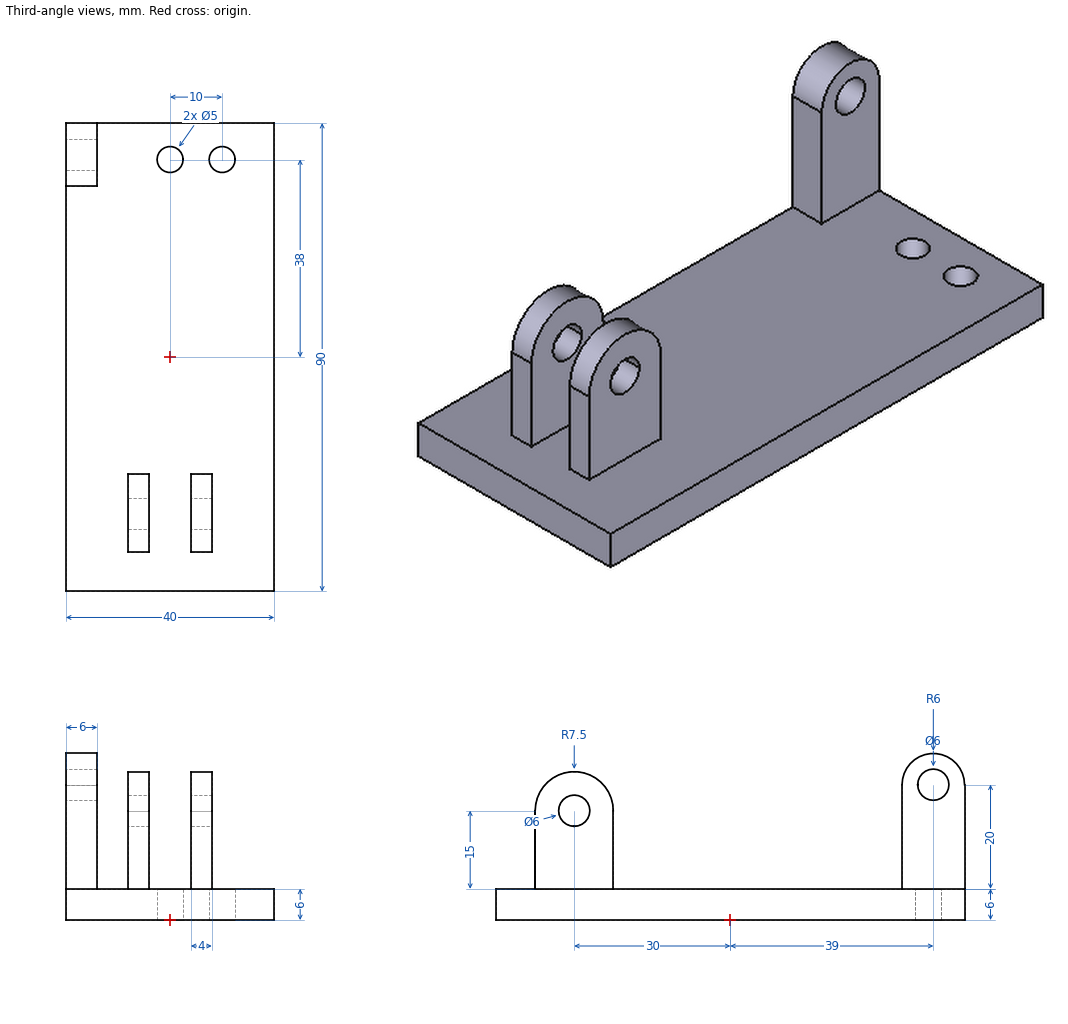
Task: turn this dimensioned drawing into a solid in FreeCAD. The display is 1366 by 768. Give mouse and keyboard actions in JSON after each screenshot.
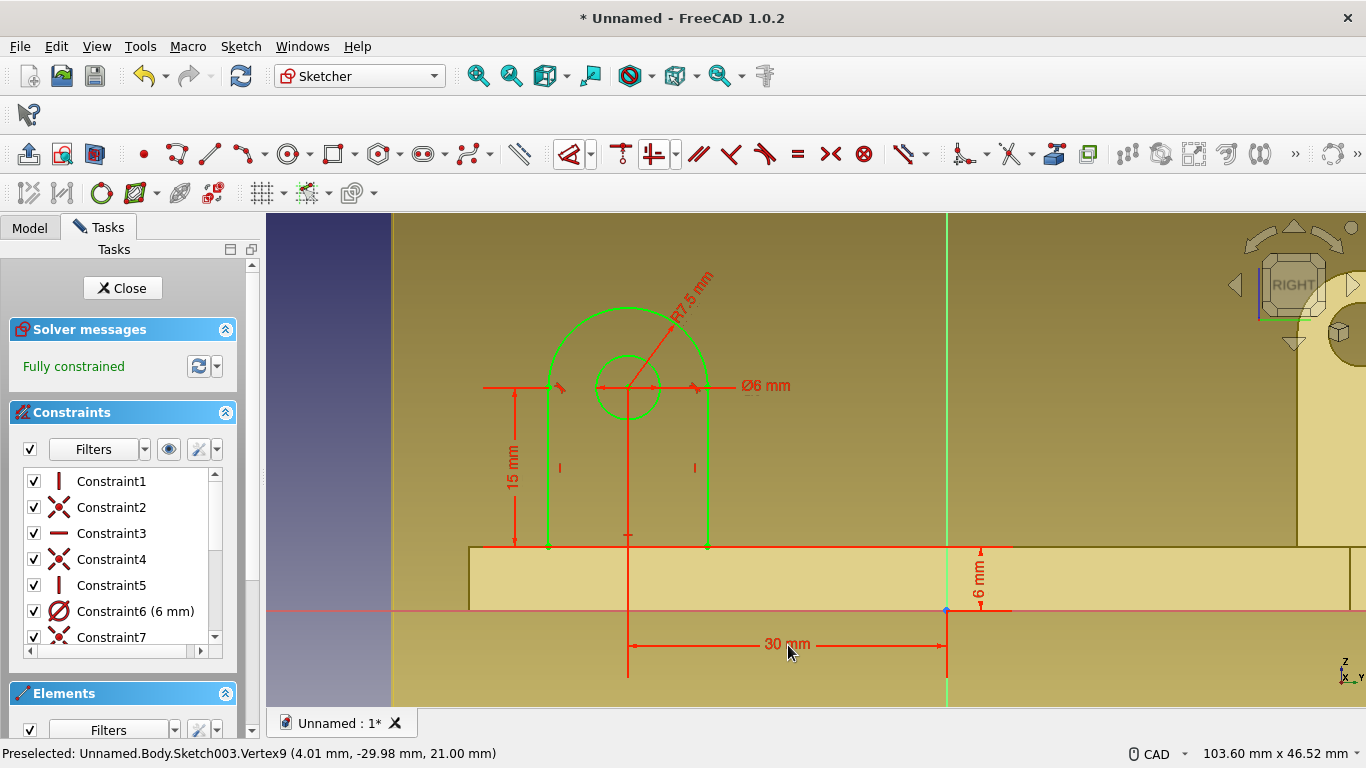
{"action": "left_click", "coordinate": [123, 288]}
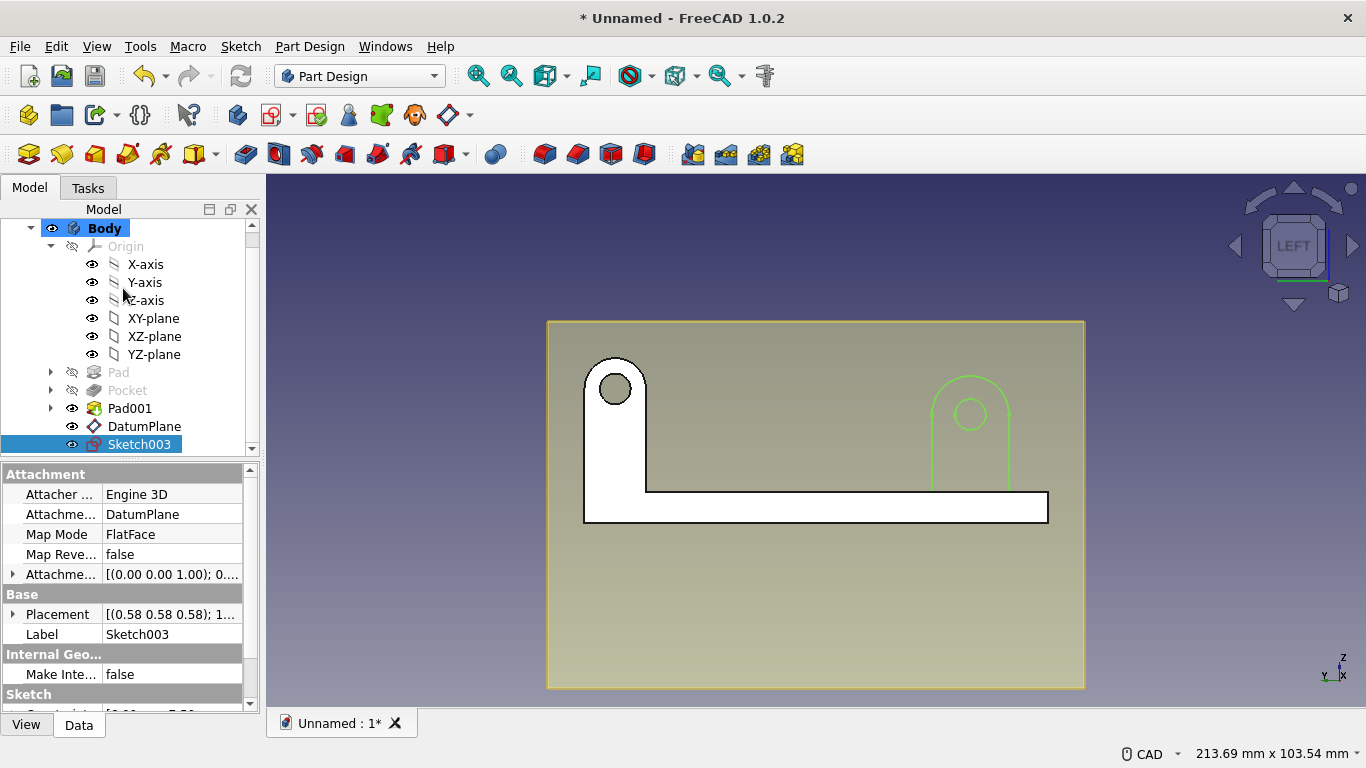
{"action": "left_click", "coordinate": [29, 154]}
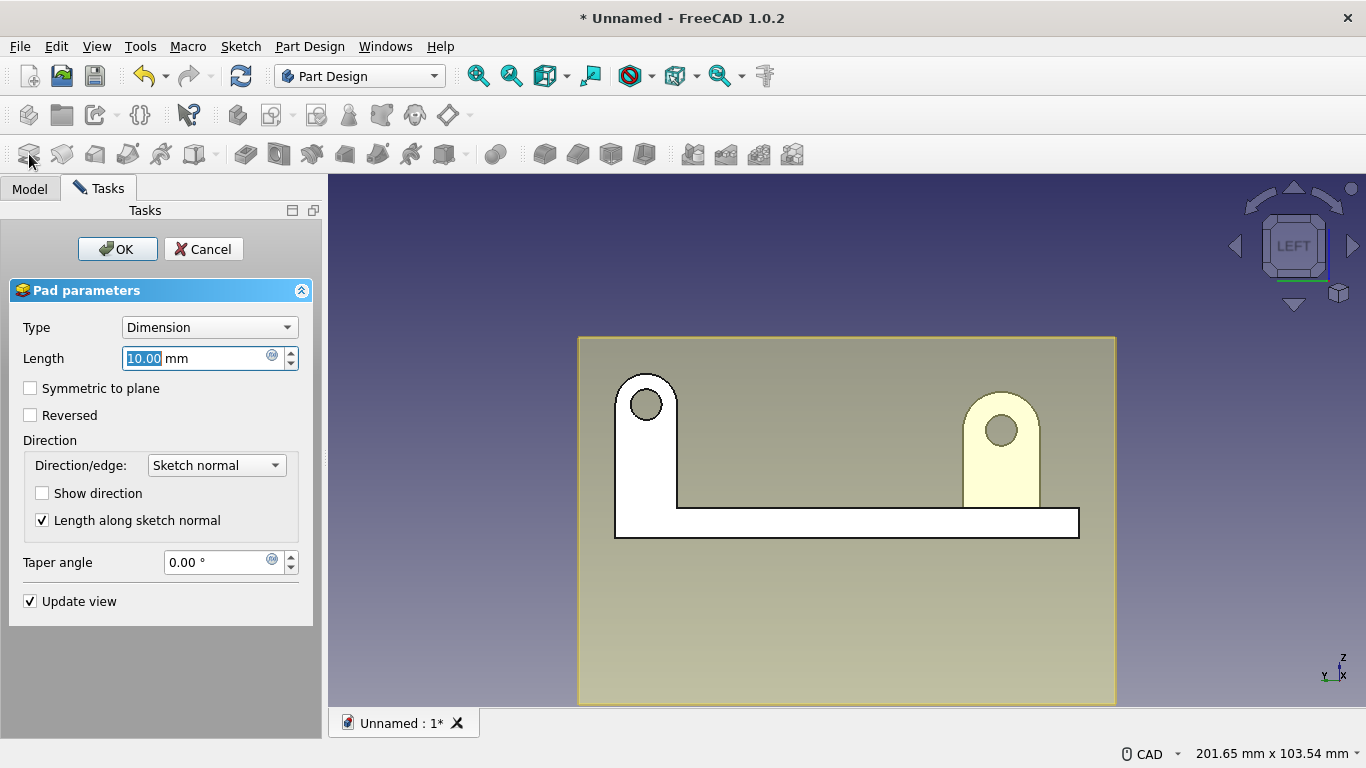
{"action": "type", "text": "4"}
{"action": "key", "text": "Tab"}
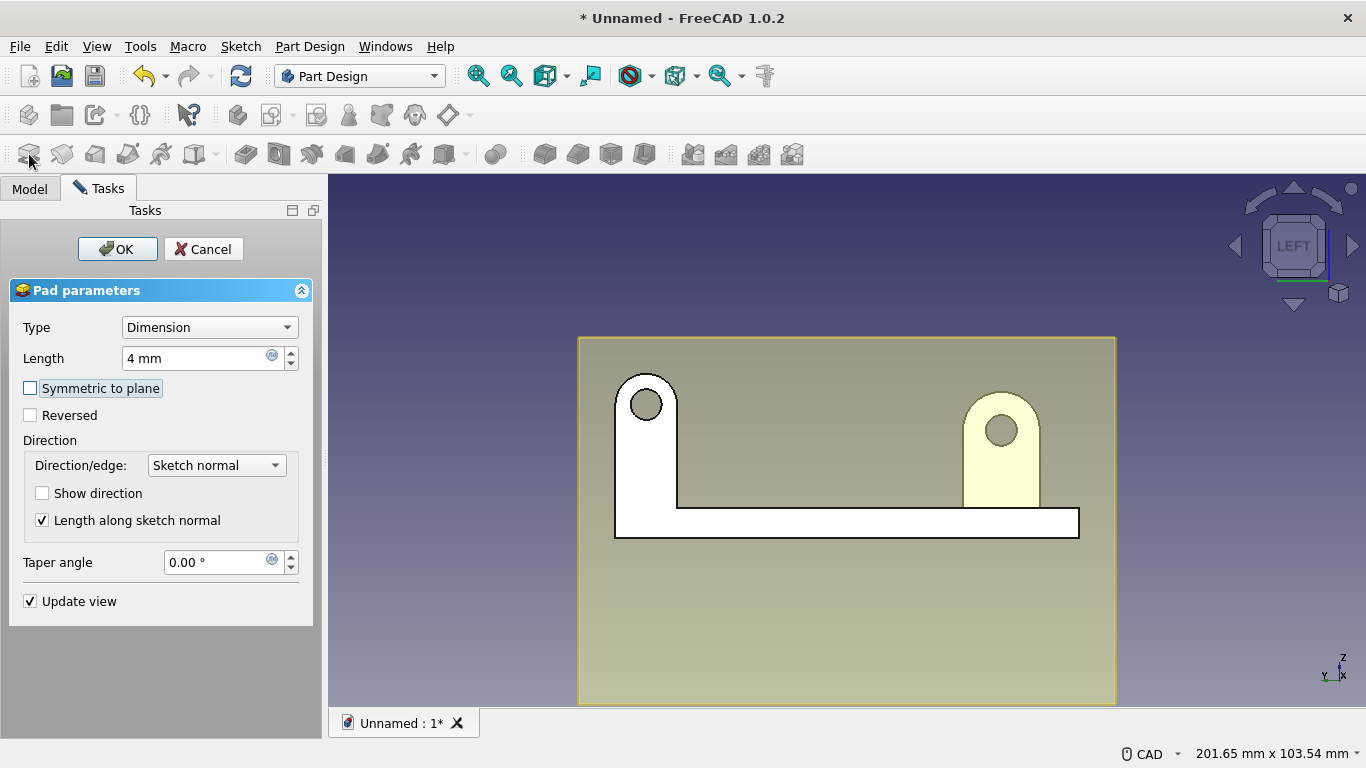
{"action": "left_click", "coordinate": [118, 249]}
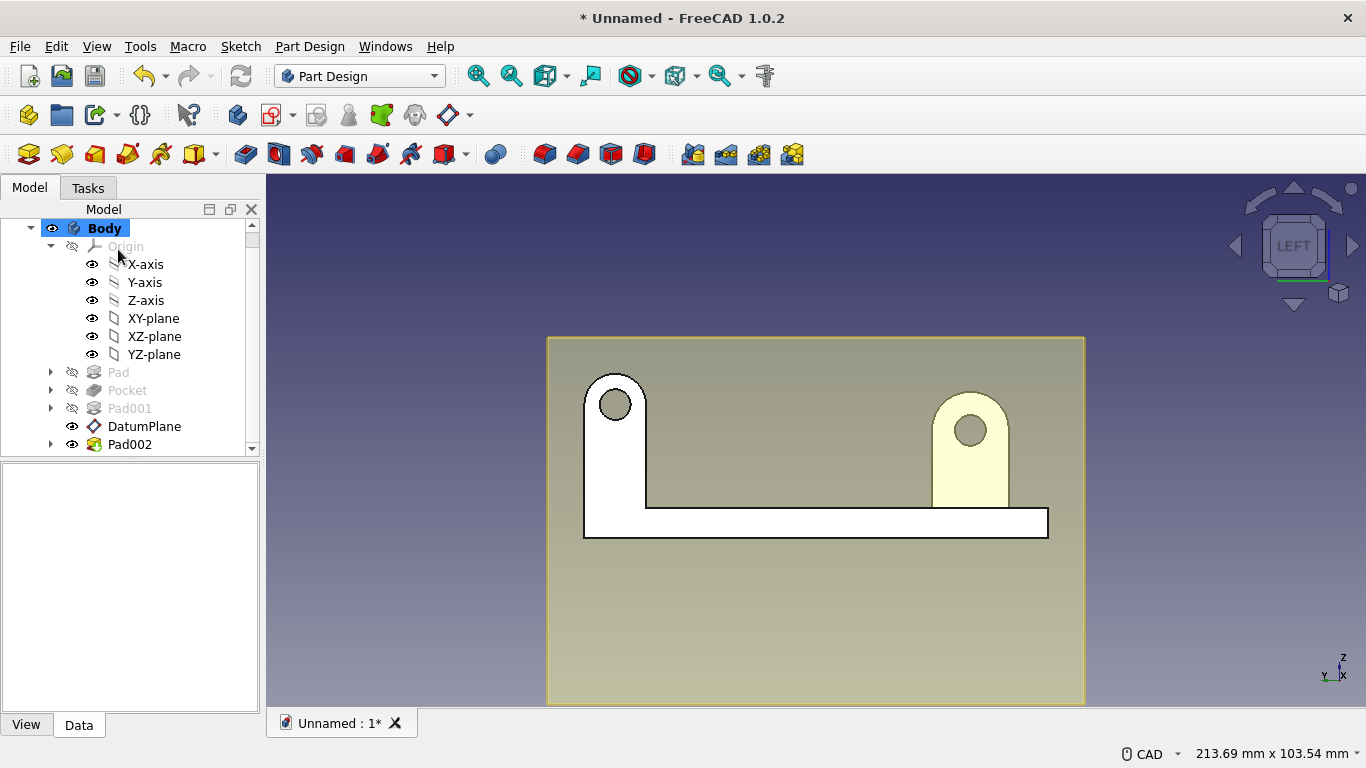
{"action": "left_click", "coordinate": [117, 426]}
{"action": "key", "text": "space"}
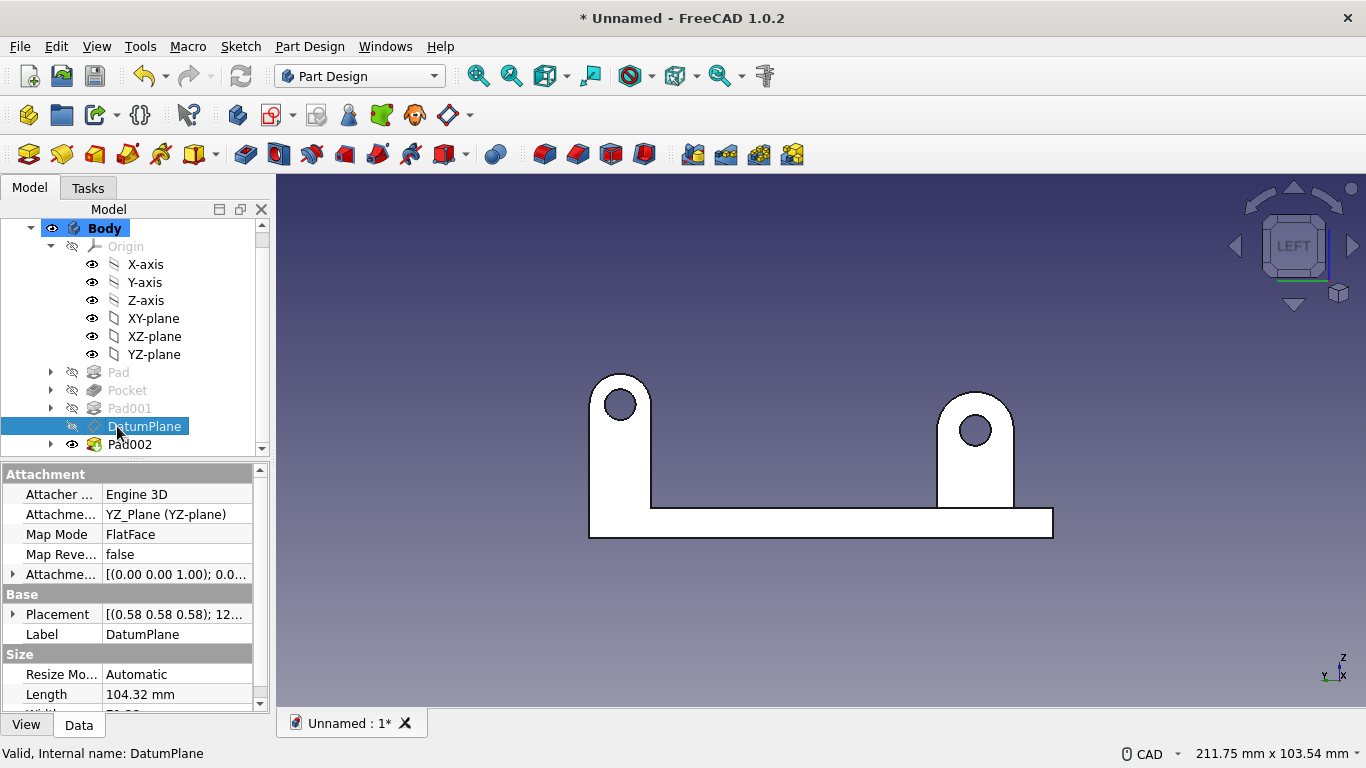
{"action": "key", "text": "v f"}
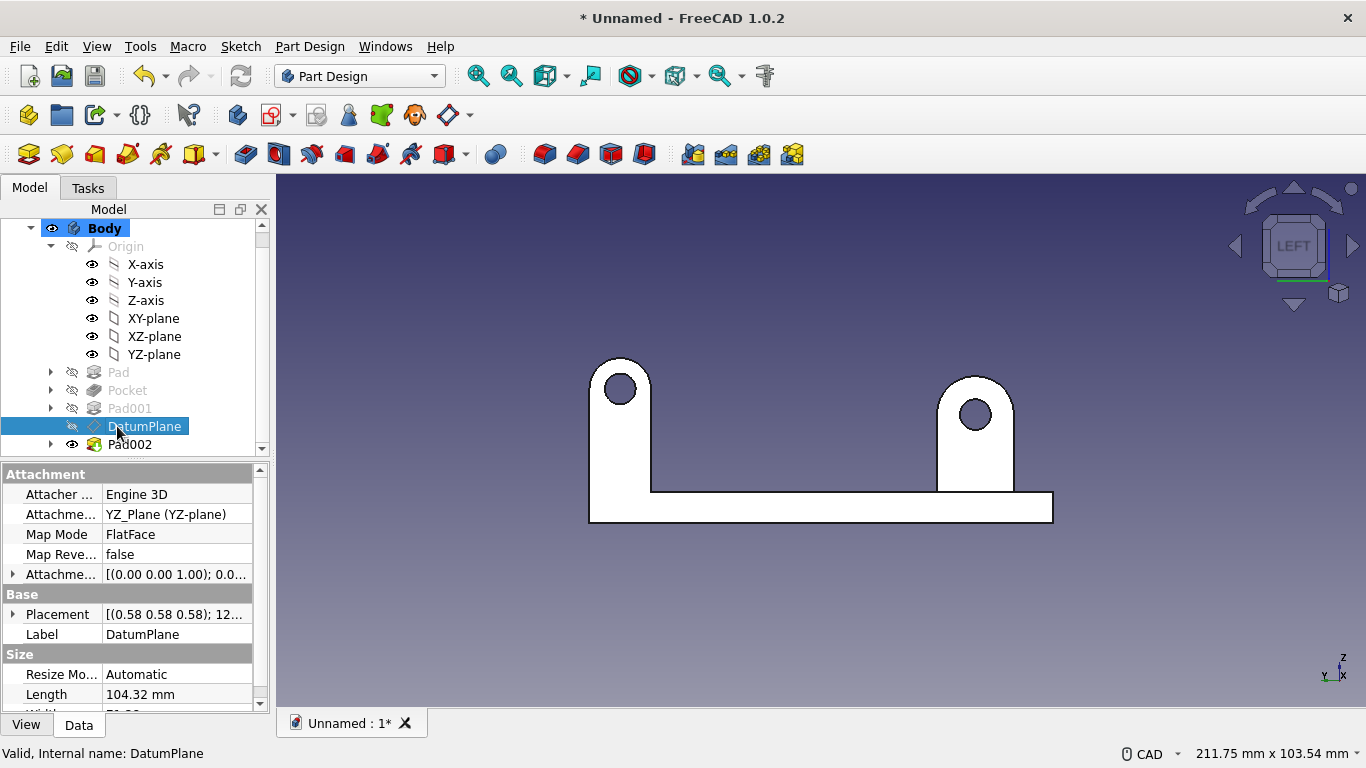
{"action": "left_click", "coordinate": [117, 444]}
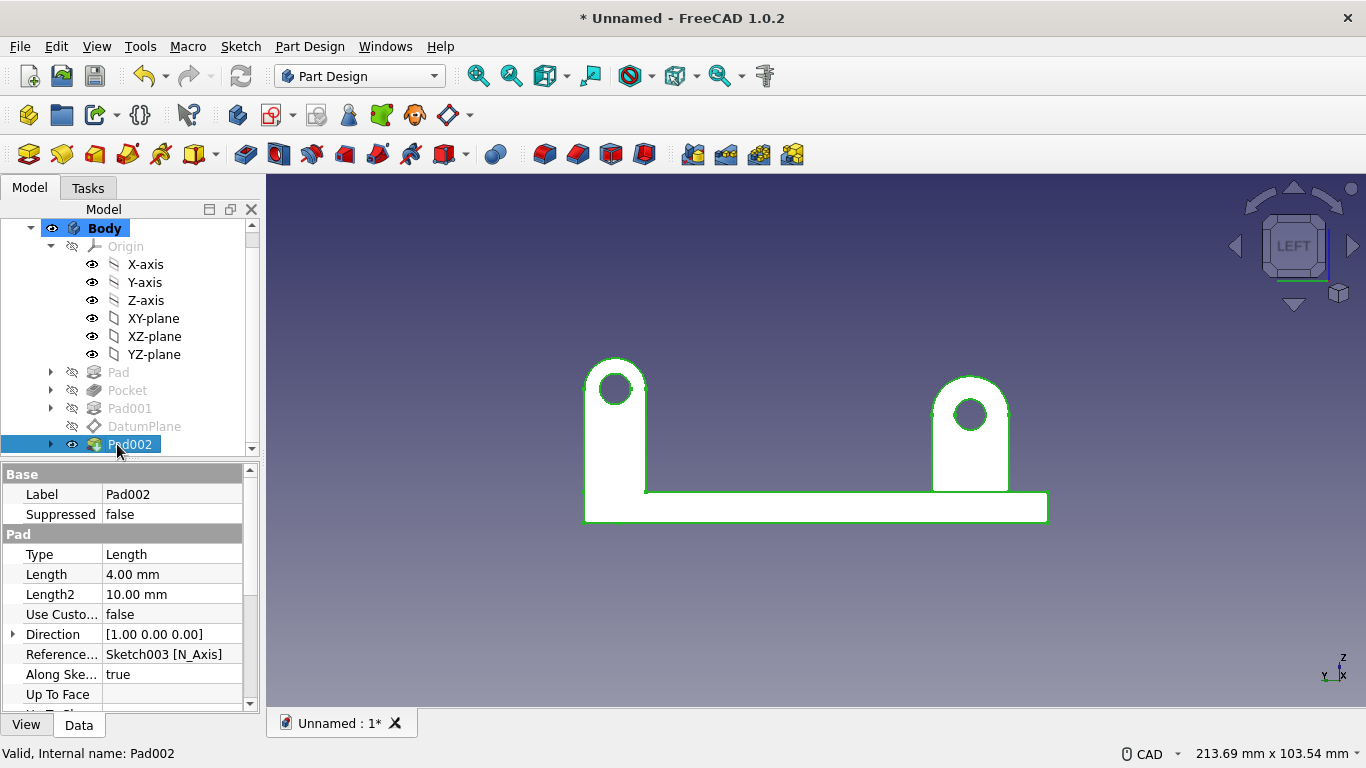
{"action": "left_click", "coordinate": [693, 154]}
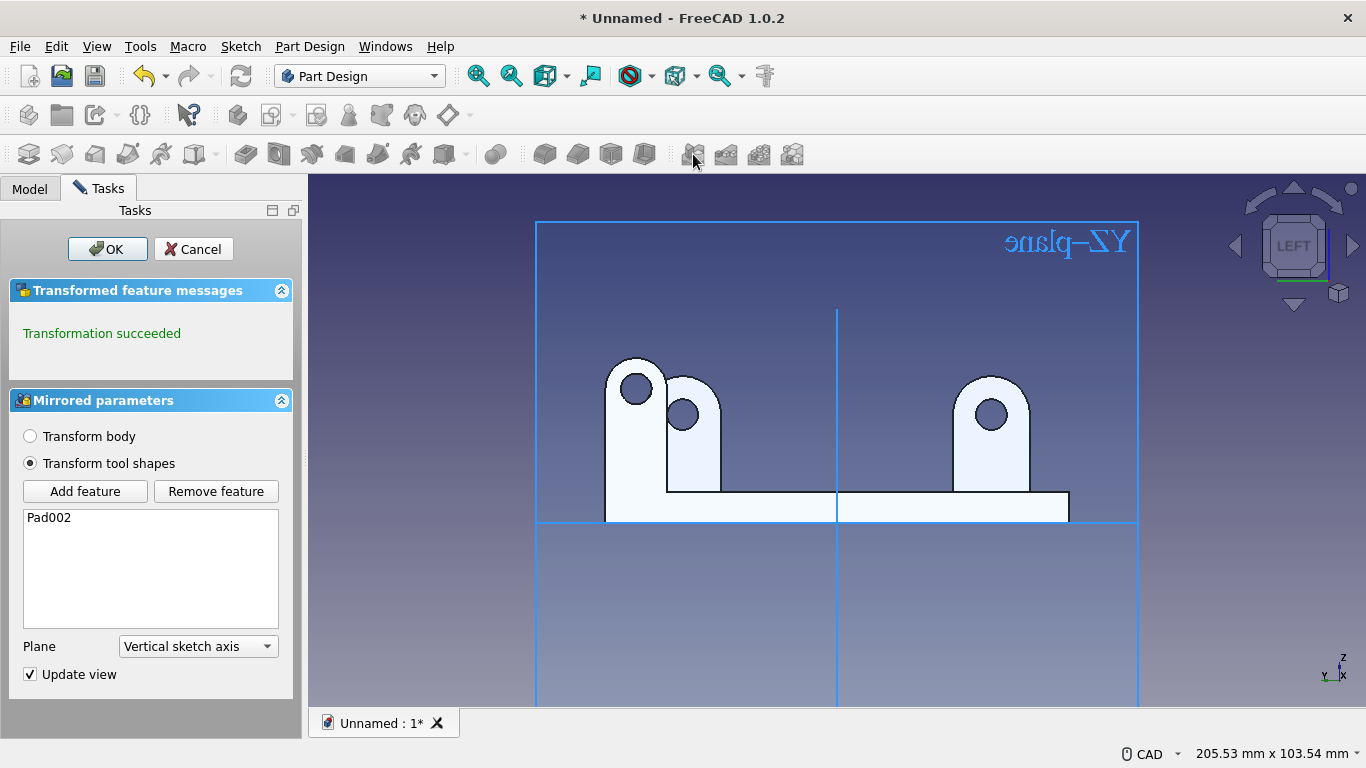
{"action": "left_click", "coordinate": [199, 646]}